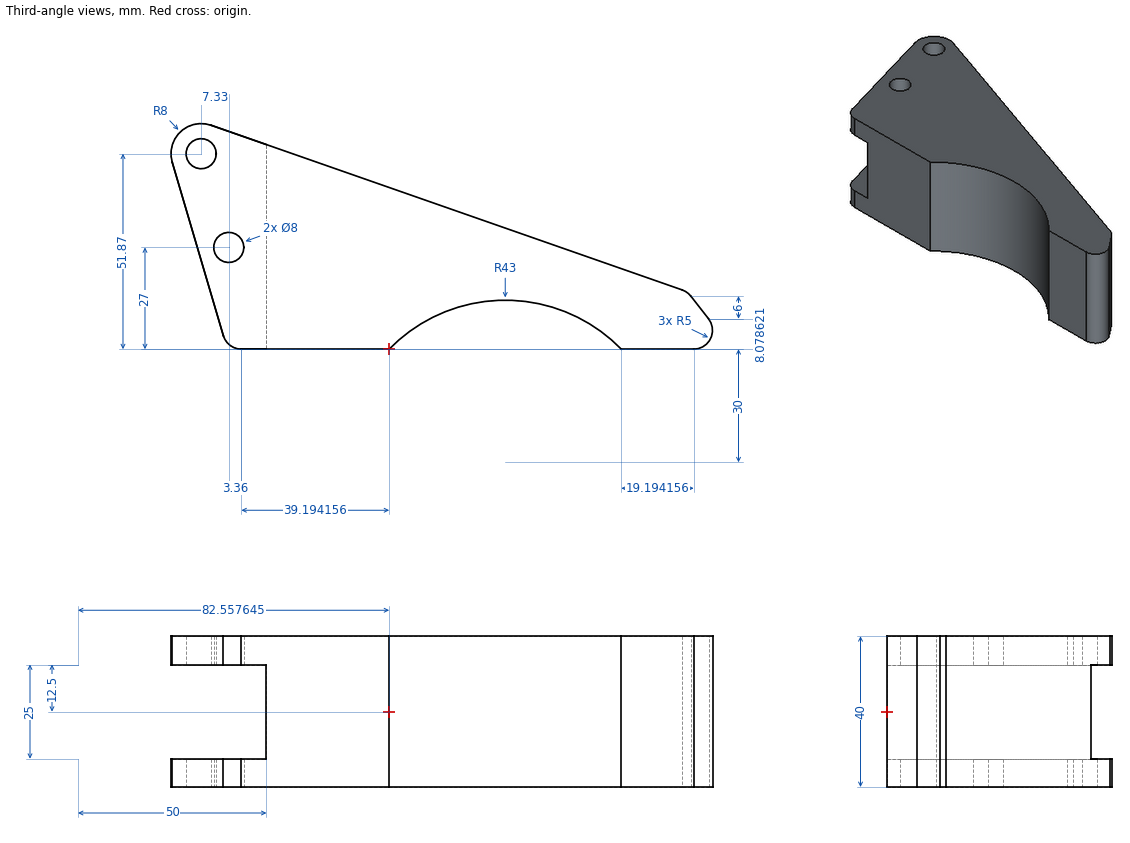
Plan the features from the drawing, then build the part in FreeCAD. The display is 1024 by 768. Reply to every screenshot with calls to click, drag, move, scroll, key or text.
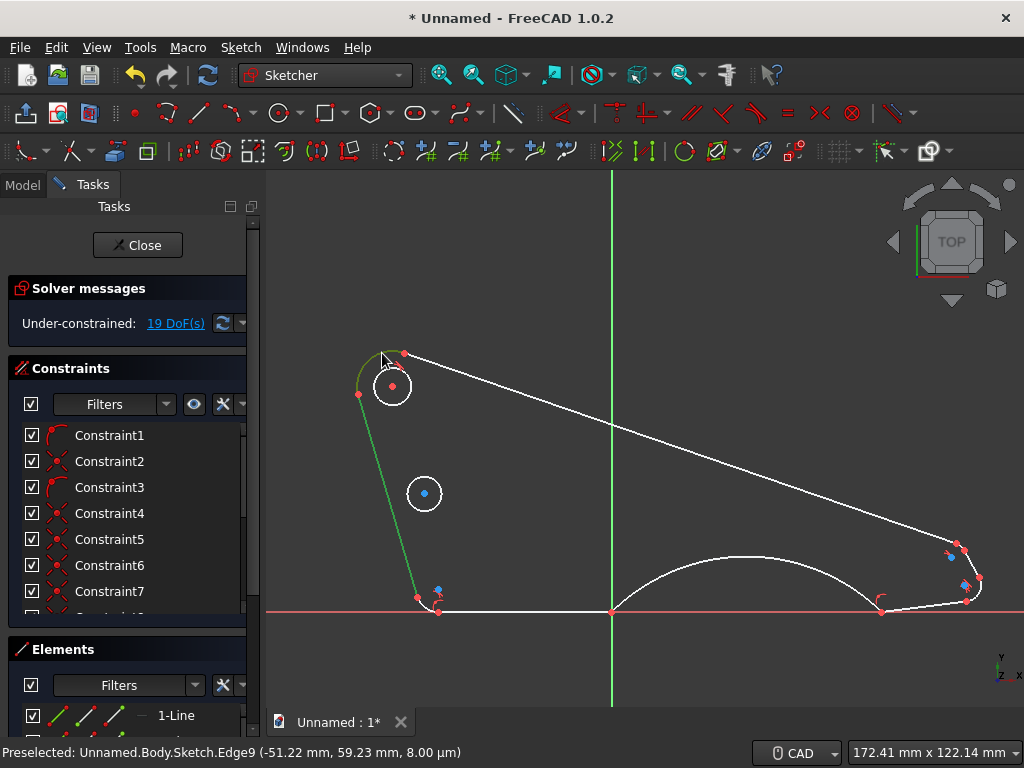
click(756, 114)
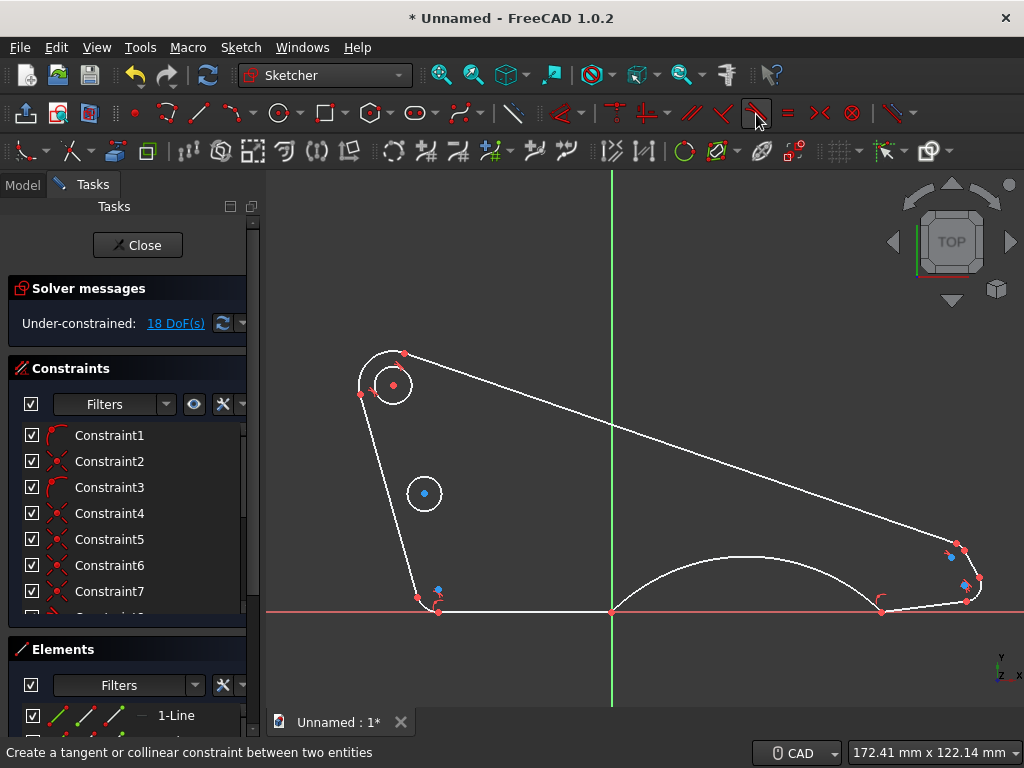
click(377, 456)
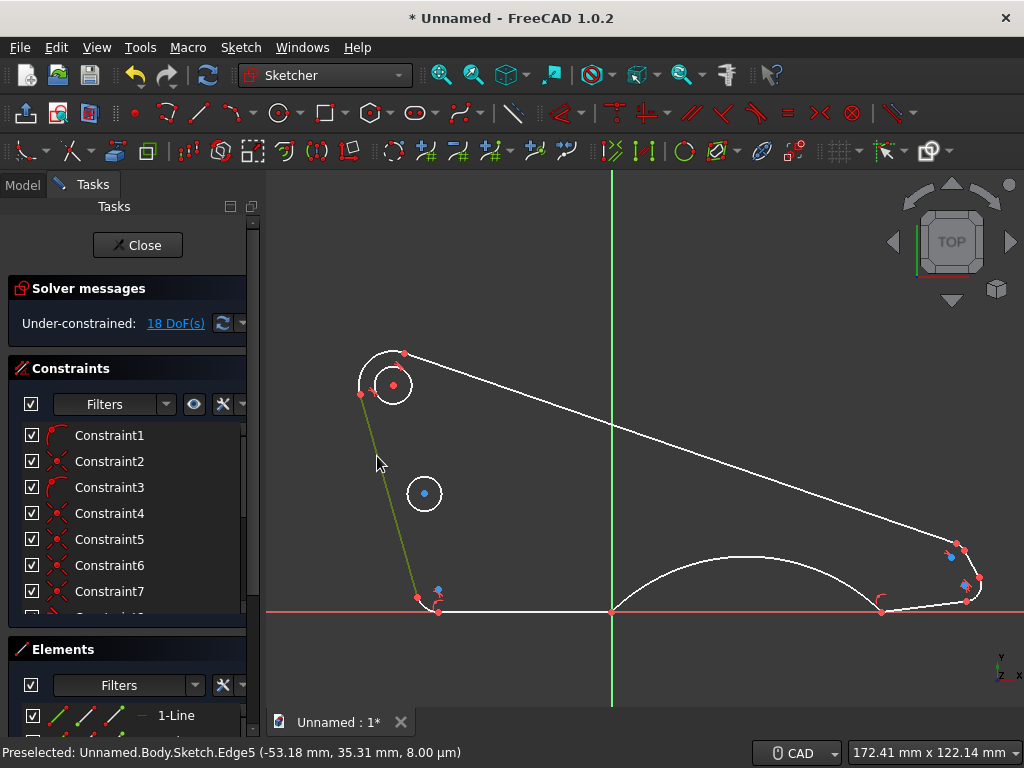
scroll(431, 611, up, 3)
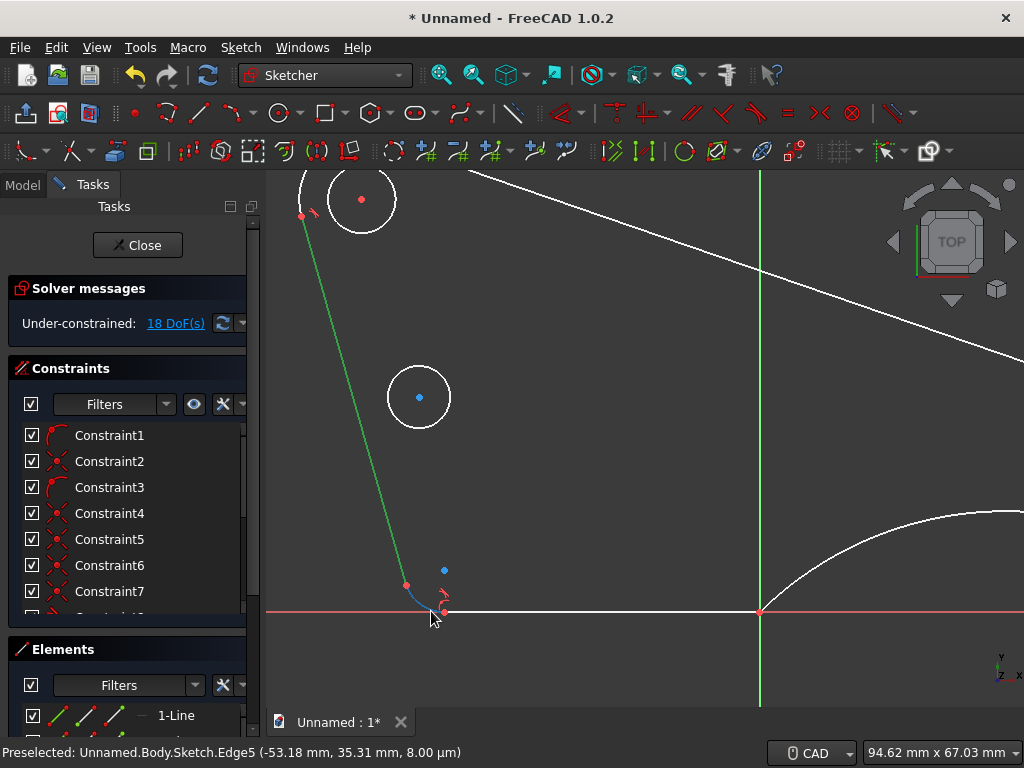
click(430, 610)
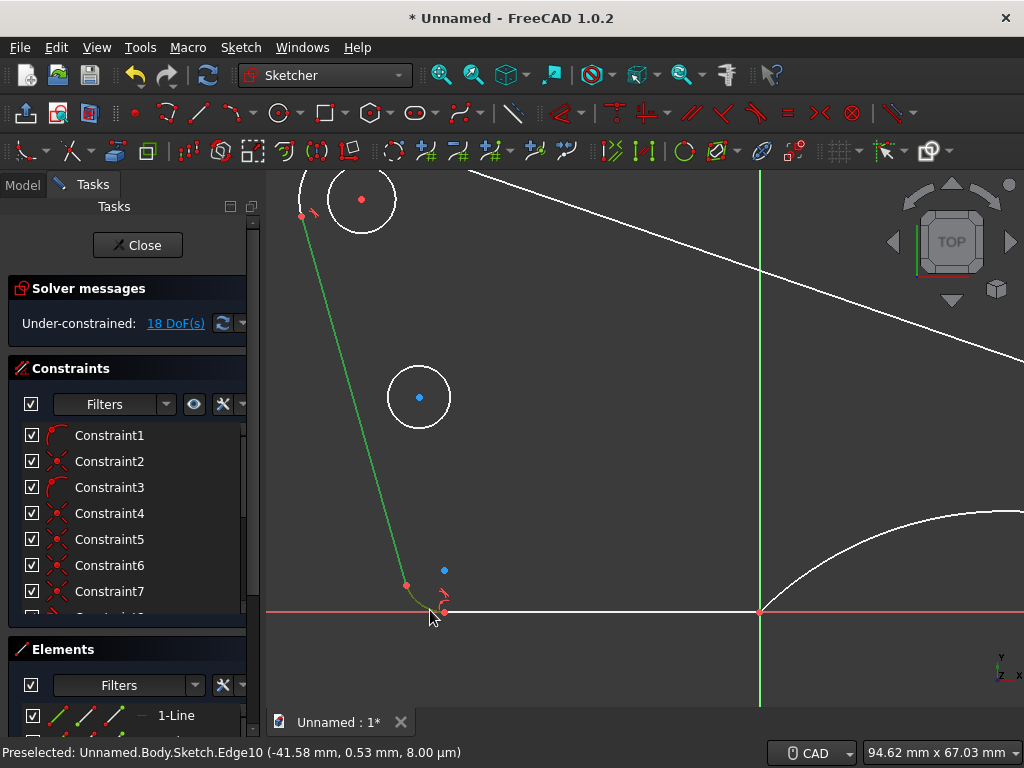
click(756, 114)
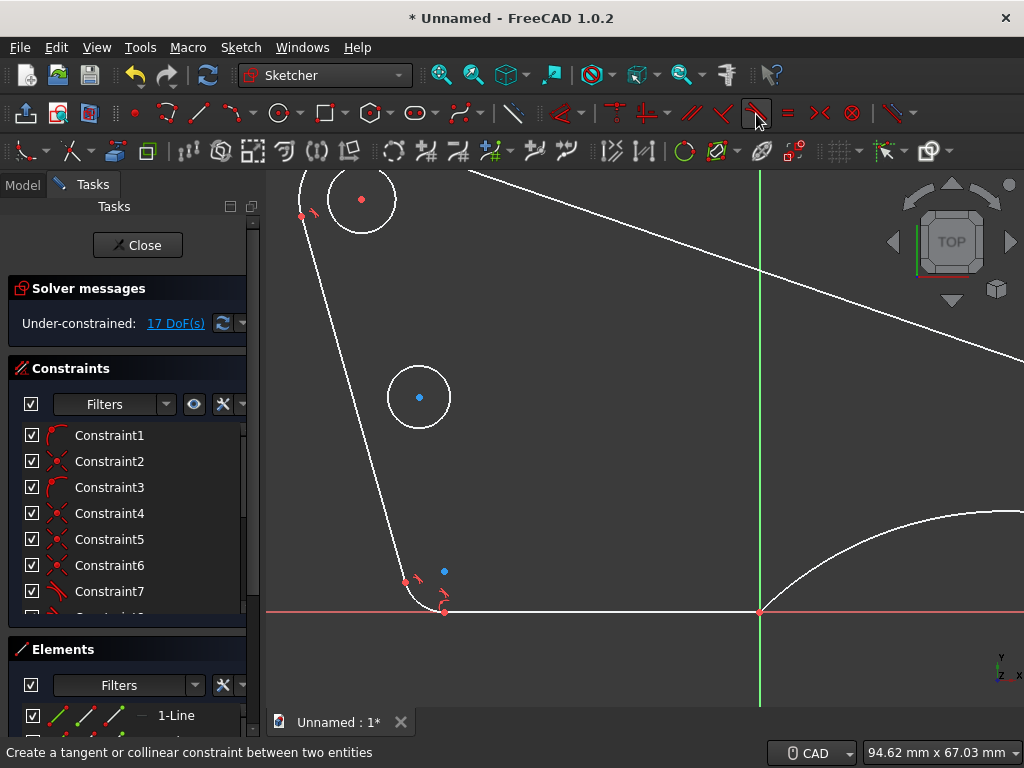
scroll(405, 476, down, 5)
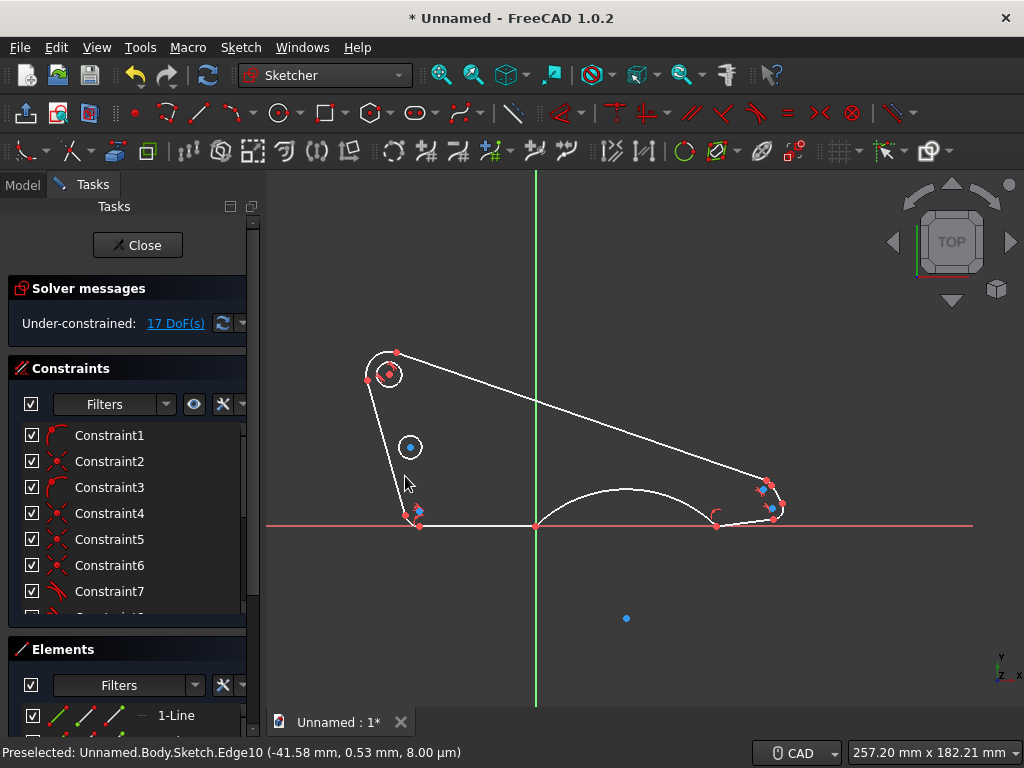
scroll(757, 521, up, 6)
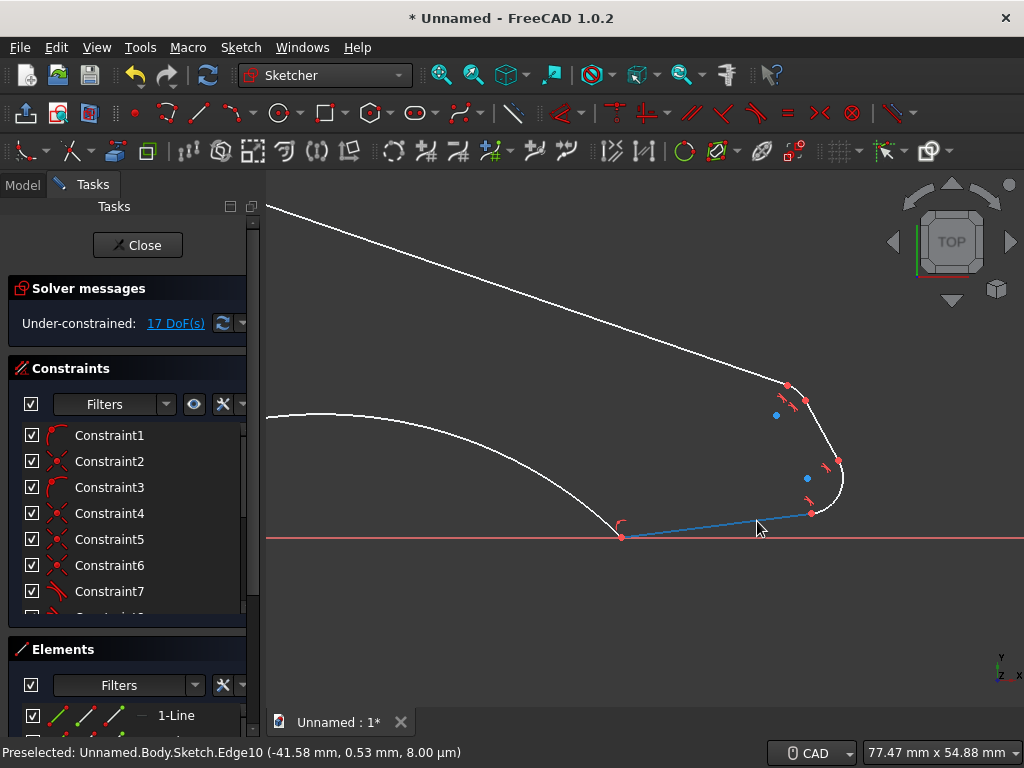
click(755, 521)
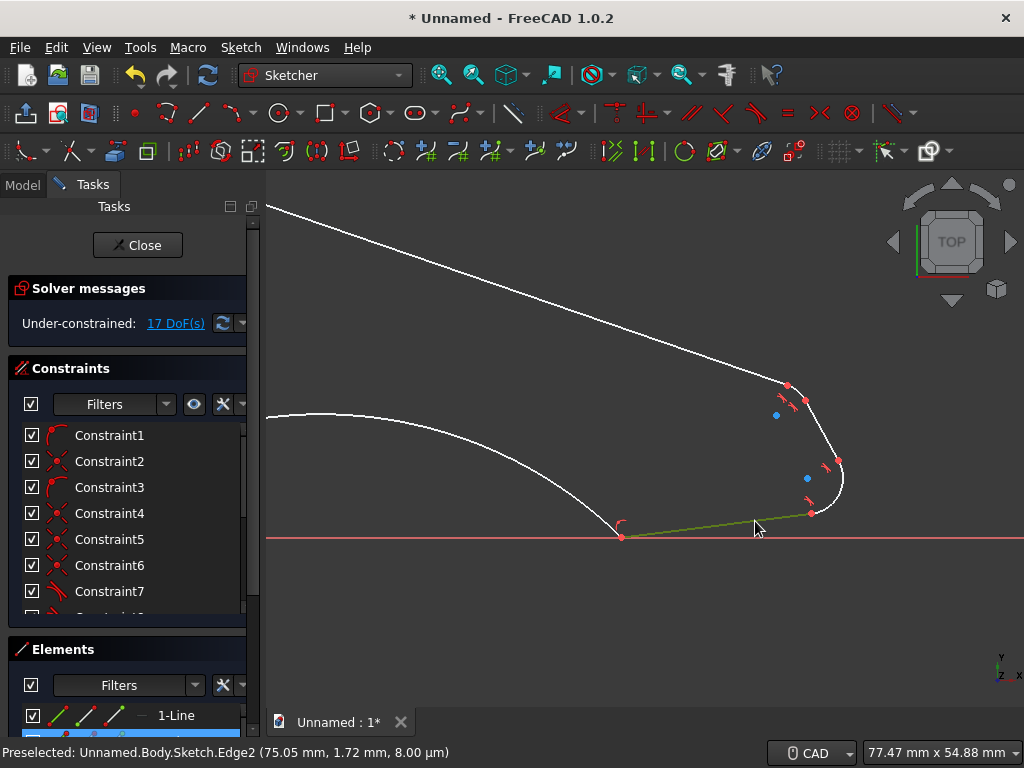
key(h)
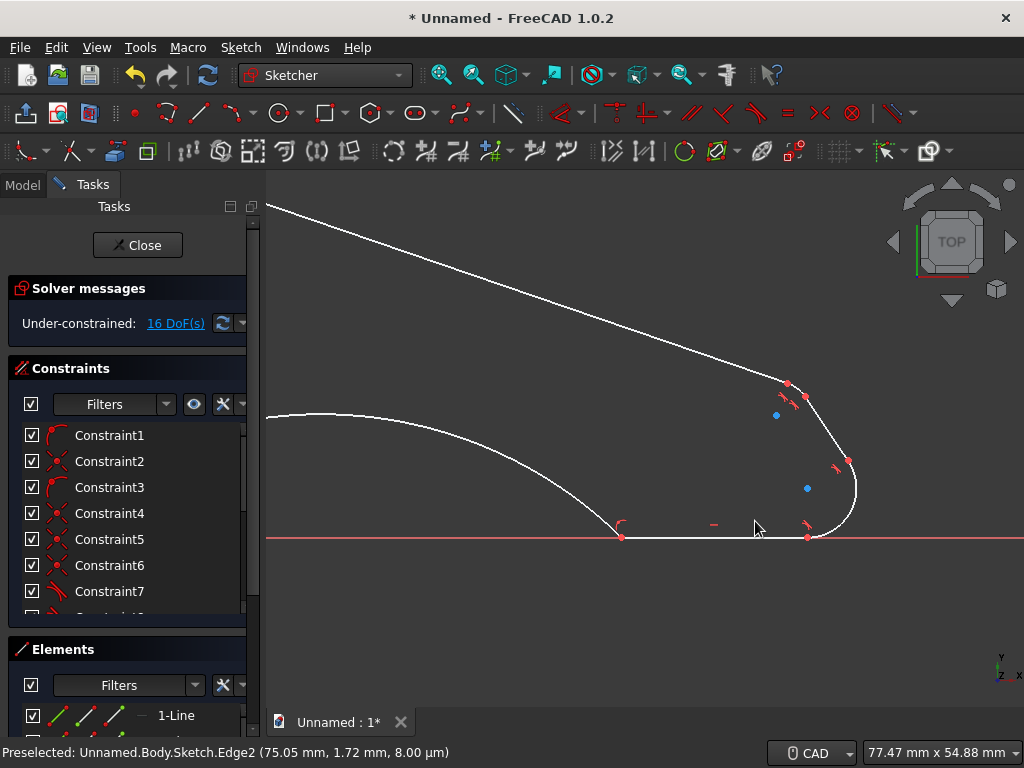
scroll(837, 528, up, 2)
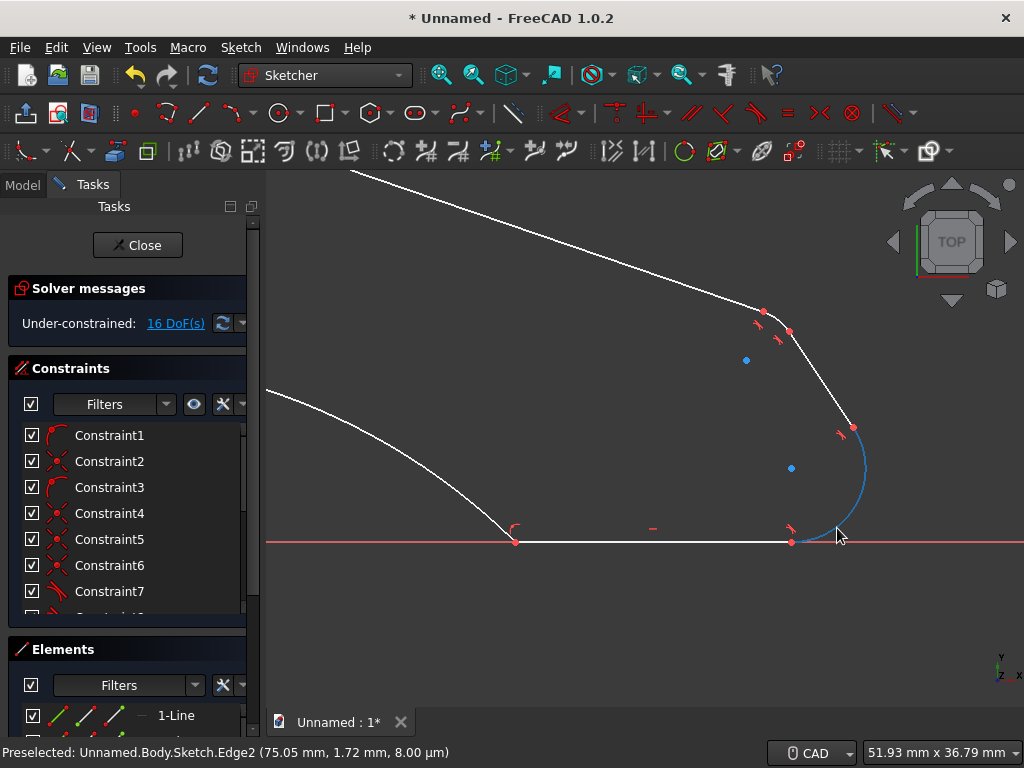
click(836, 527)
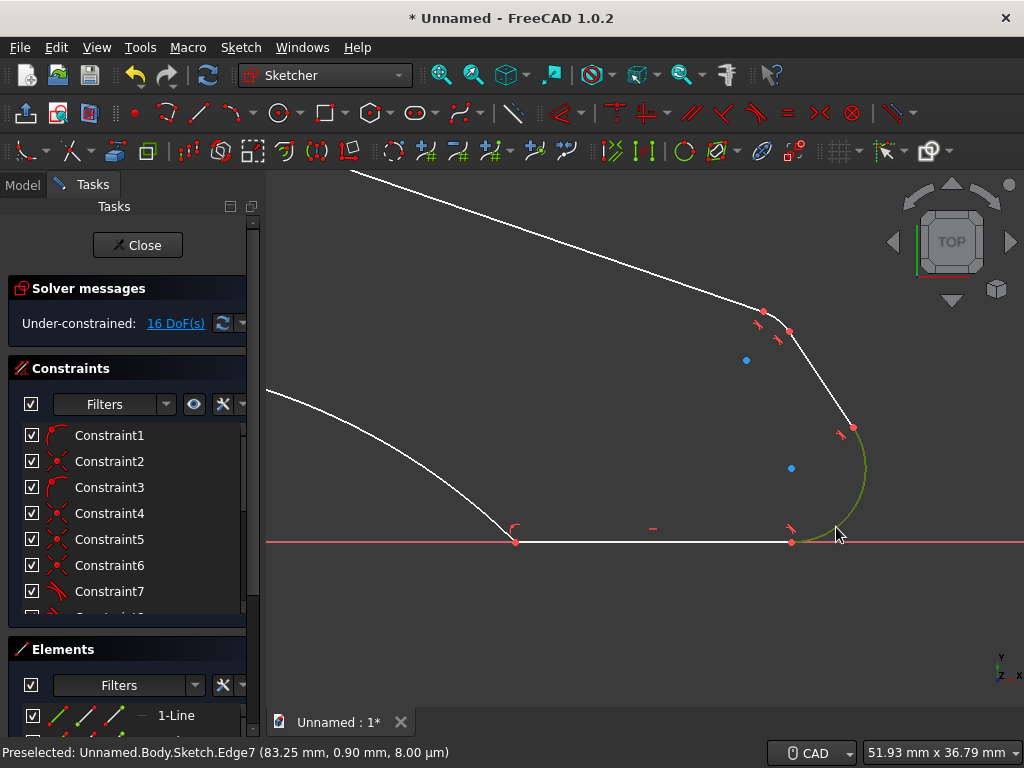
scroll(783, 324, up, 2)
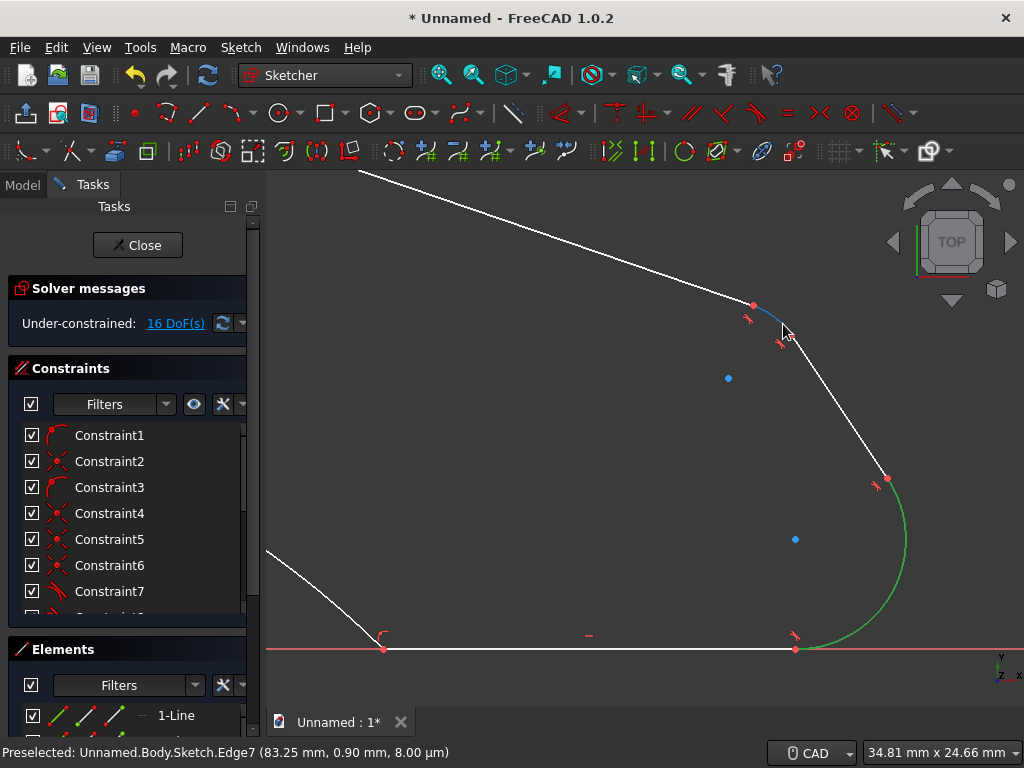
click(782, 324)